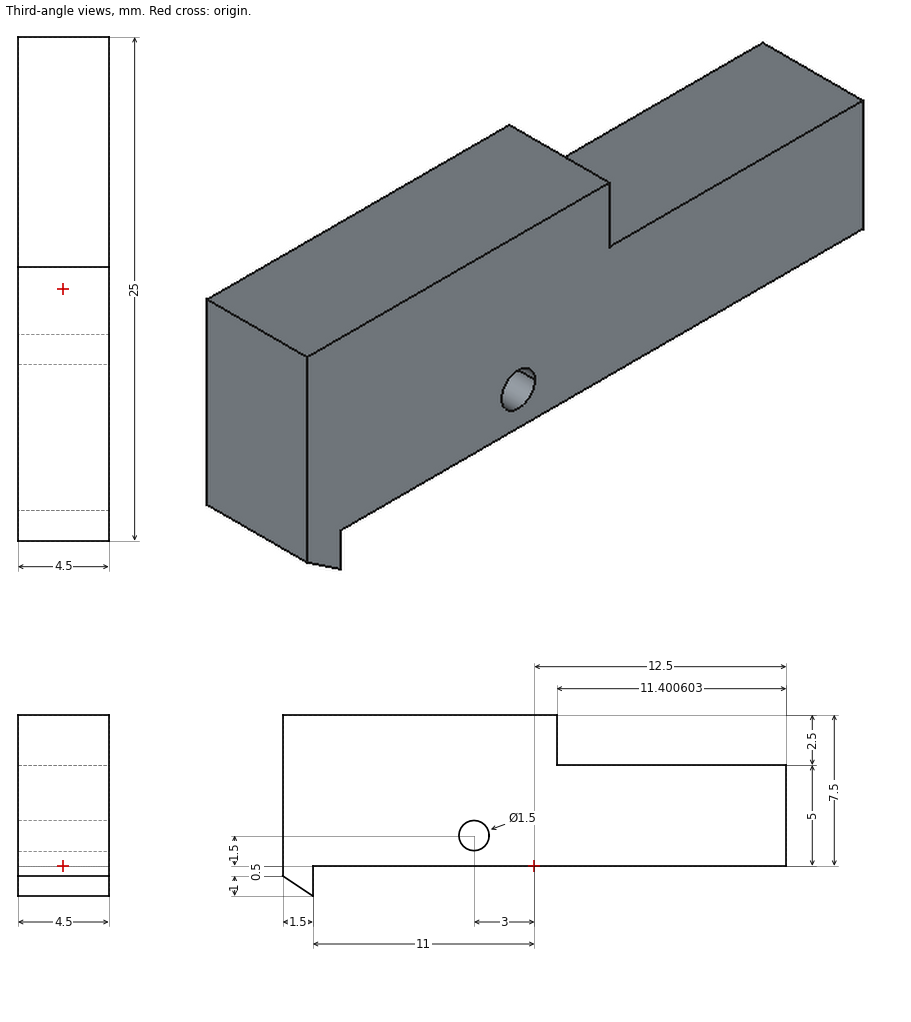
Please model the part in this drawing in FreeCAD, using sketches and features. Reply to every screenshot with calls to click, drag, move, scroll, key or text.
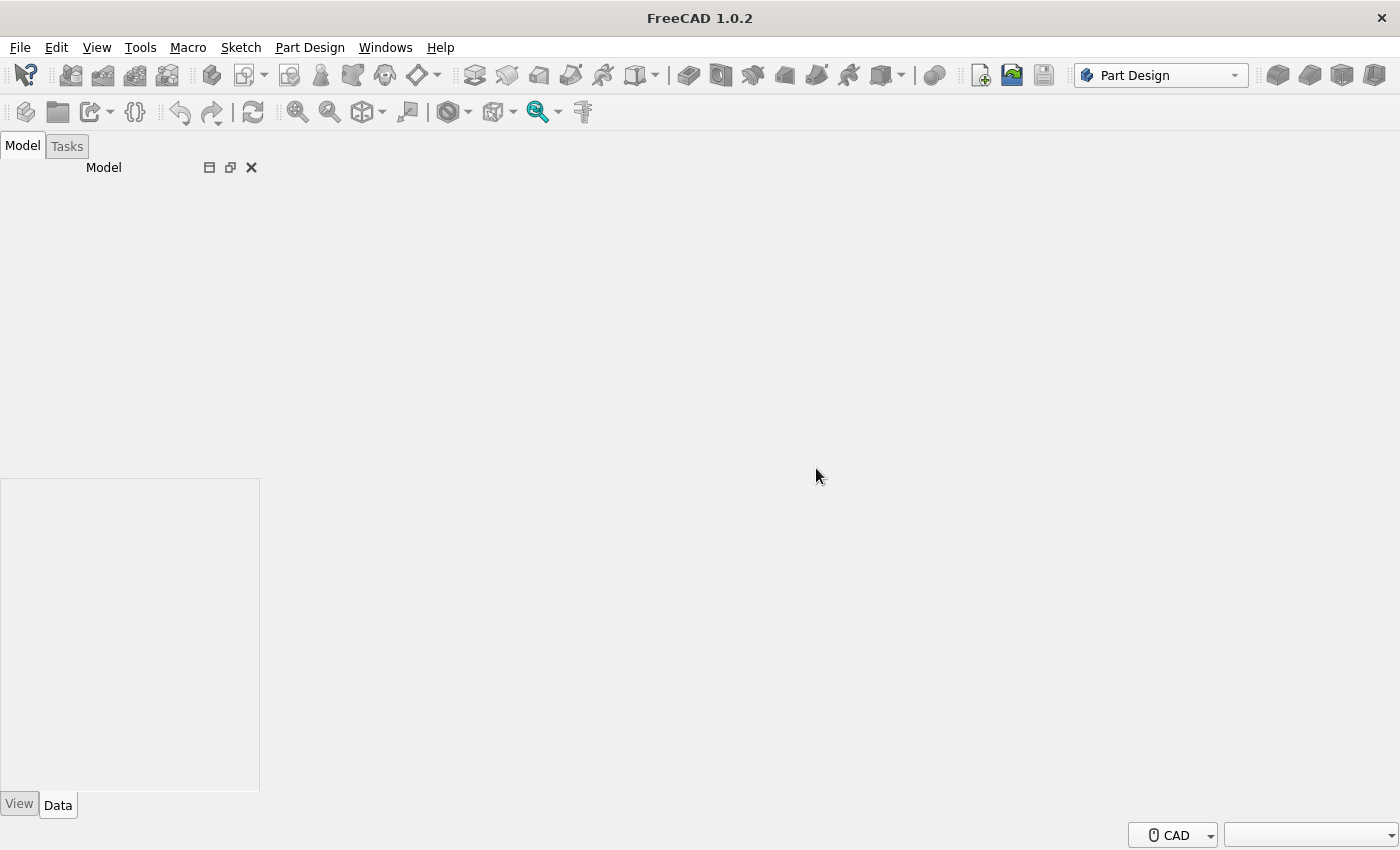
key(ctrl+n)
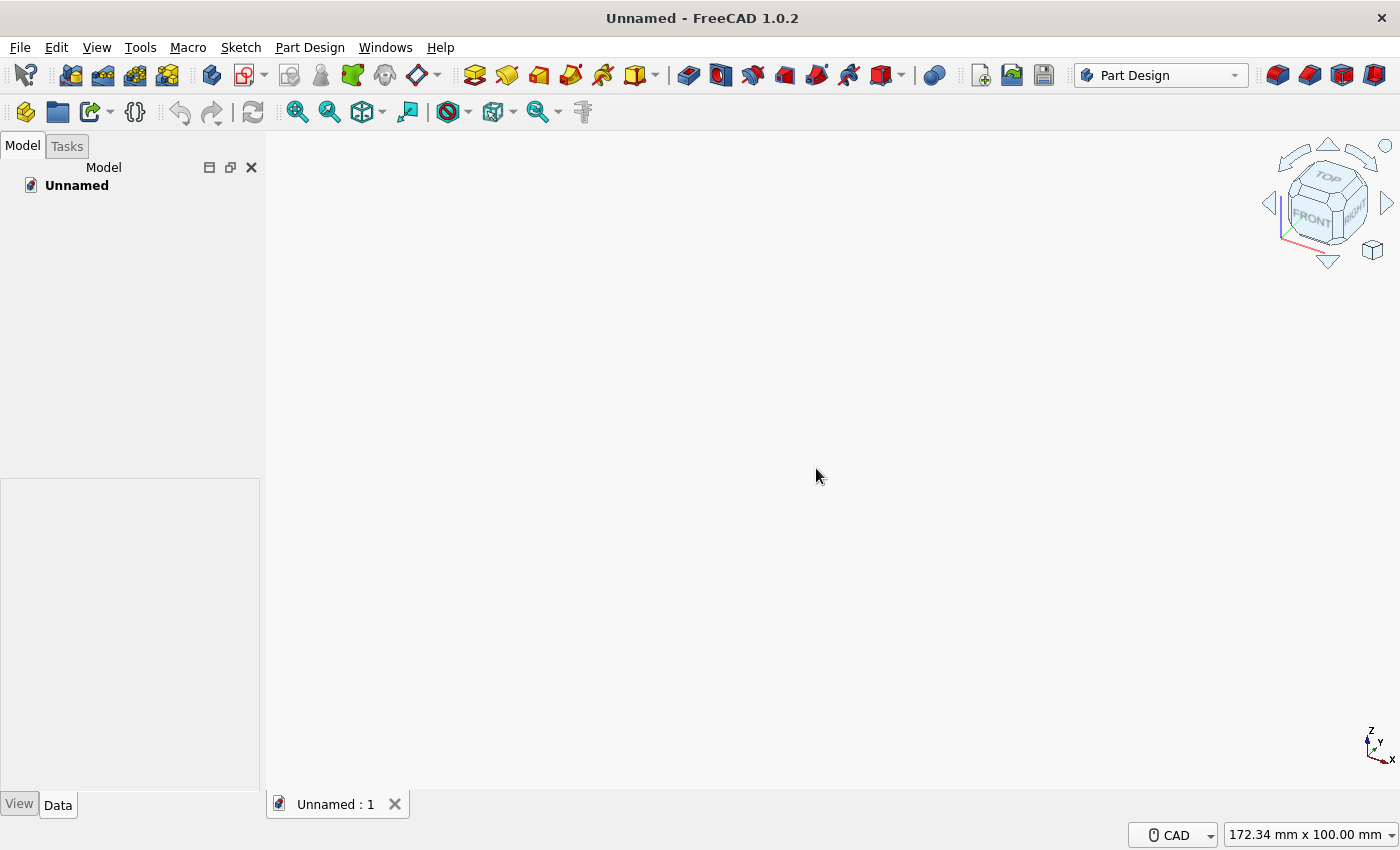
click(244, 76)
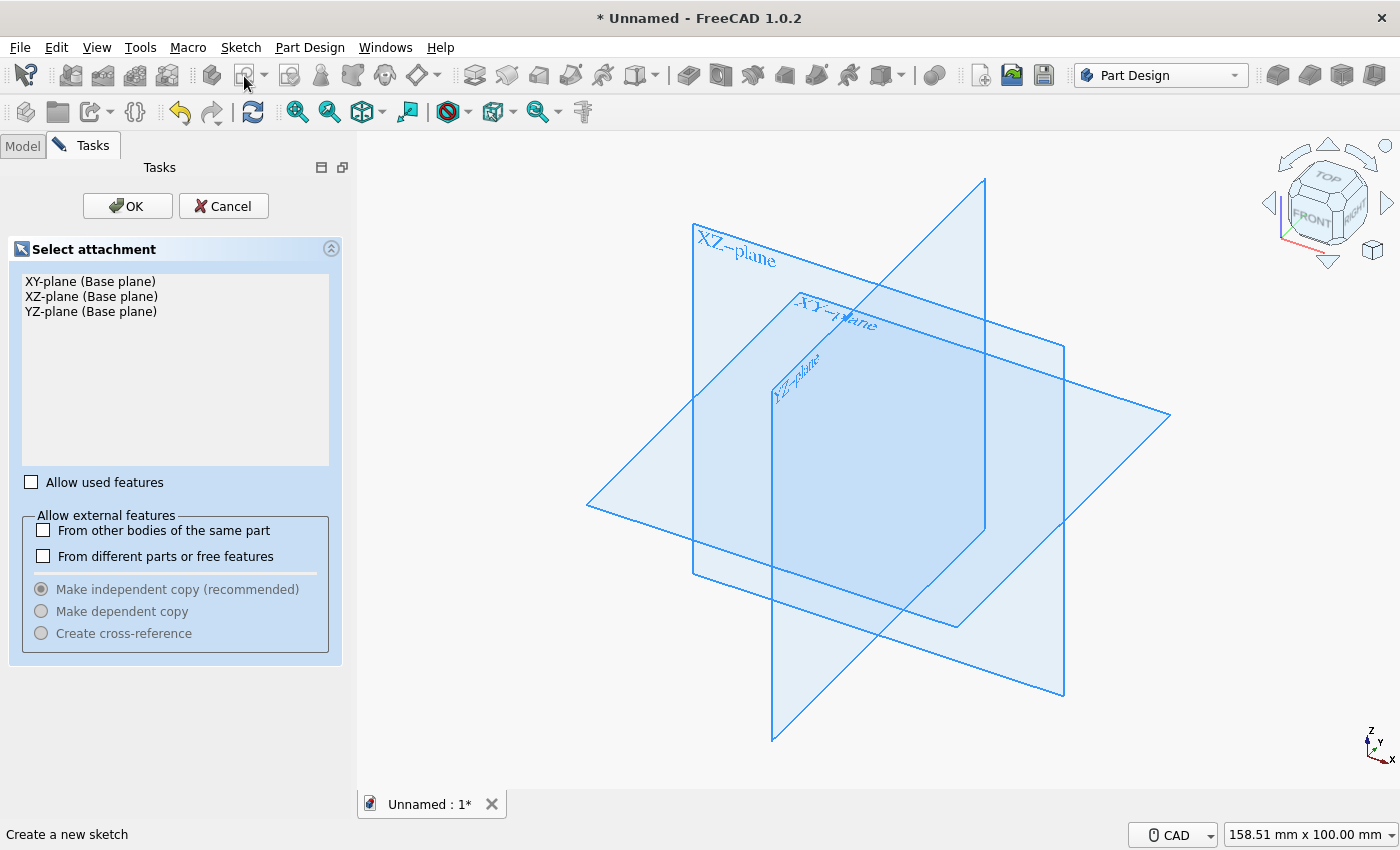
click(82, 282)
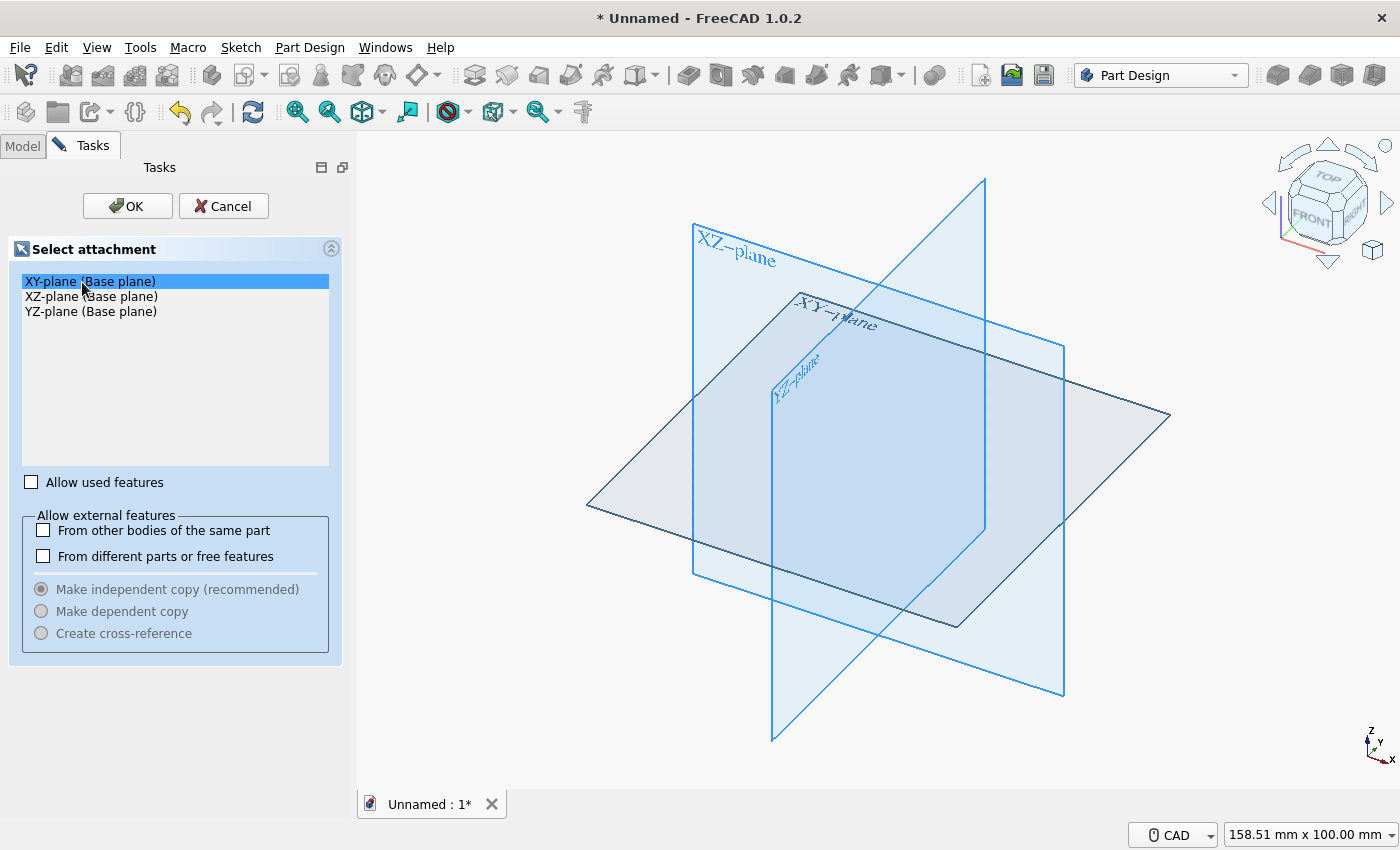
click(128, 206)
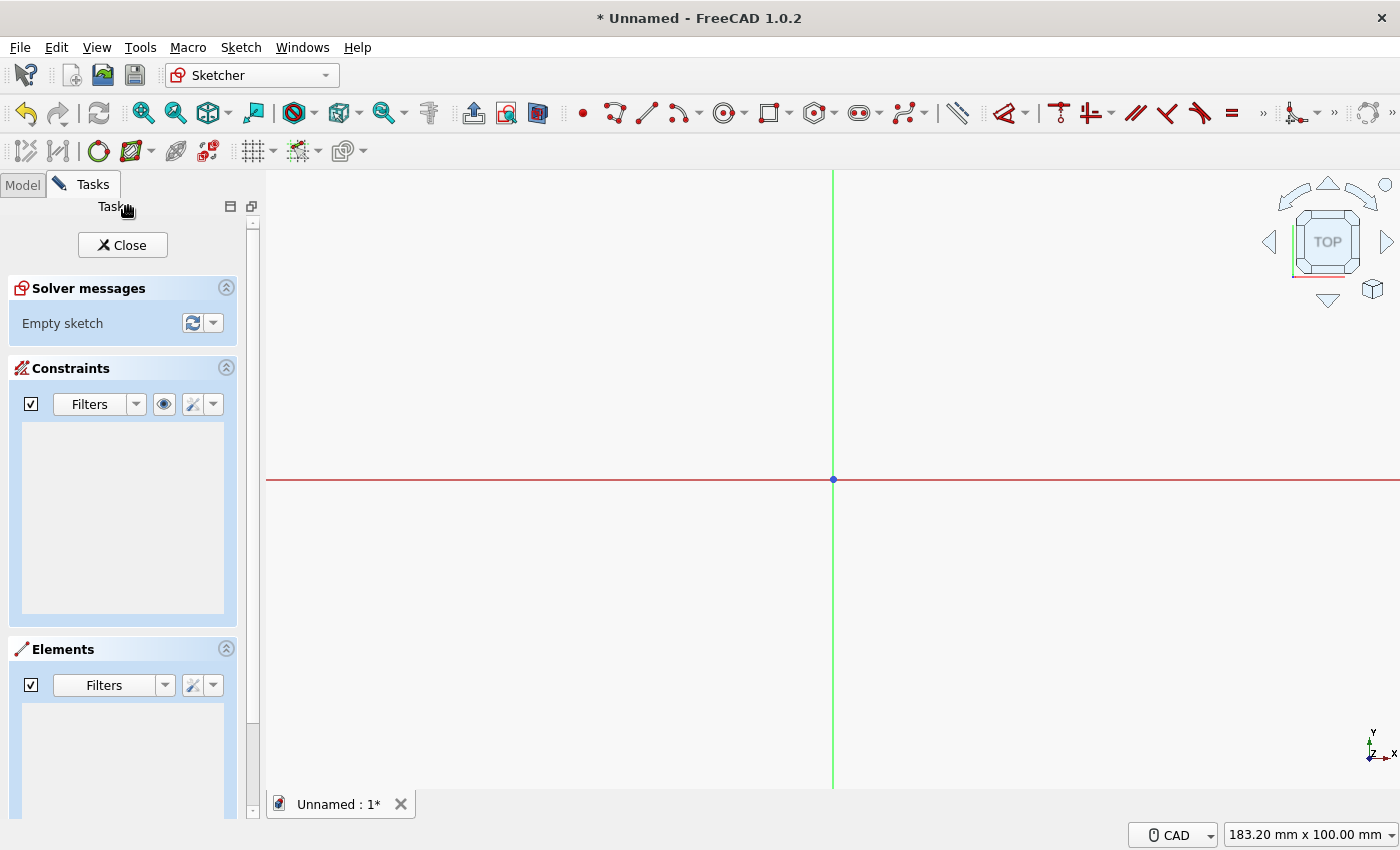
scroll(873, 480, up, 5)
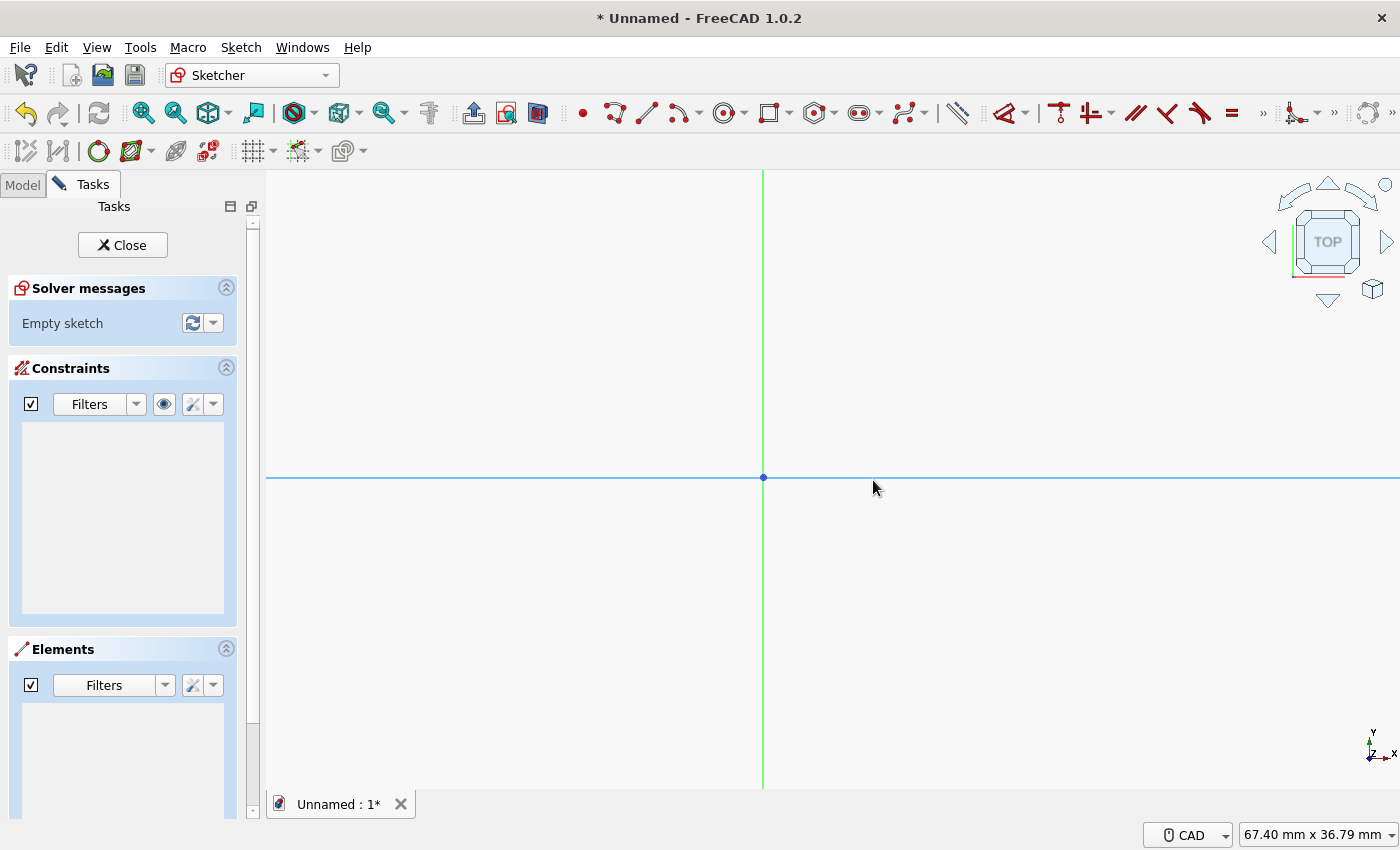
key(g)
key(v)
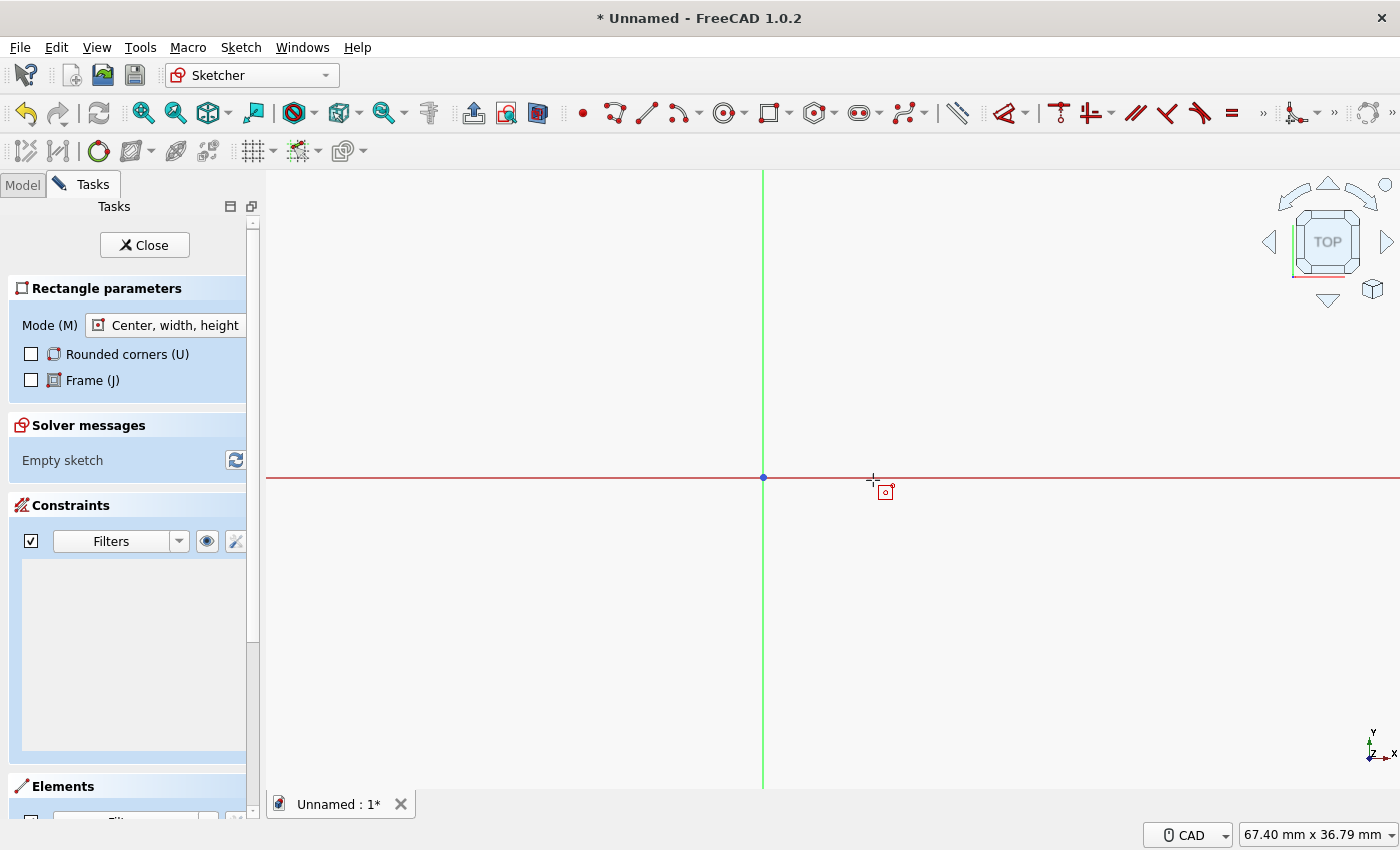
click(763, 478)
move(801, 267)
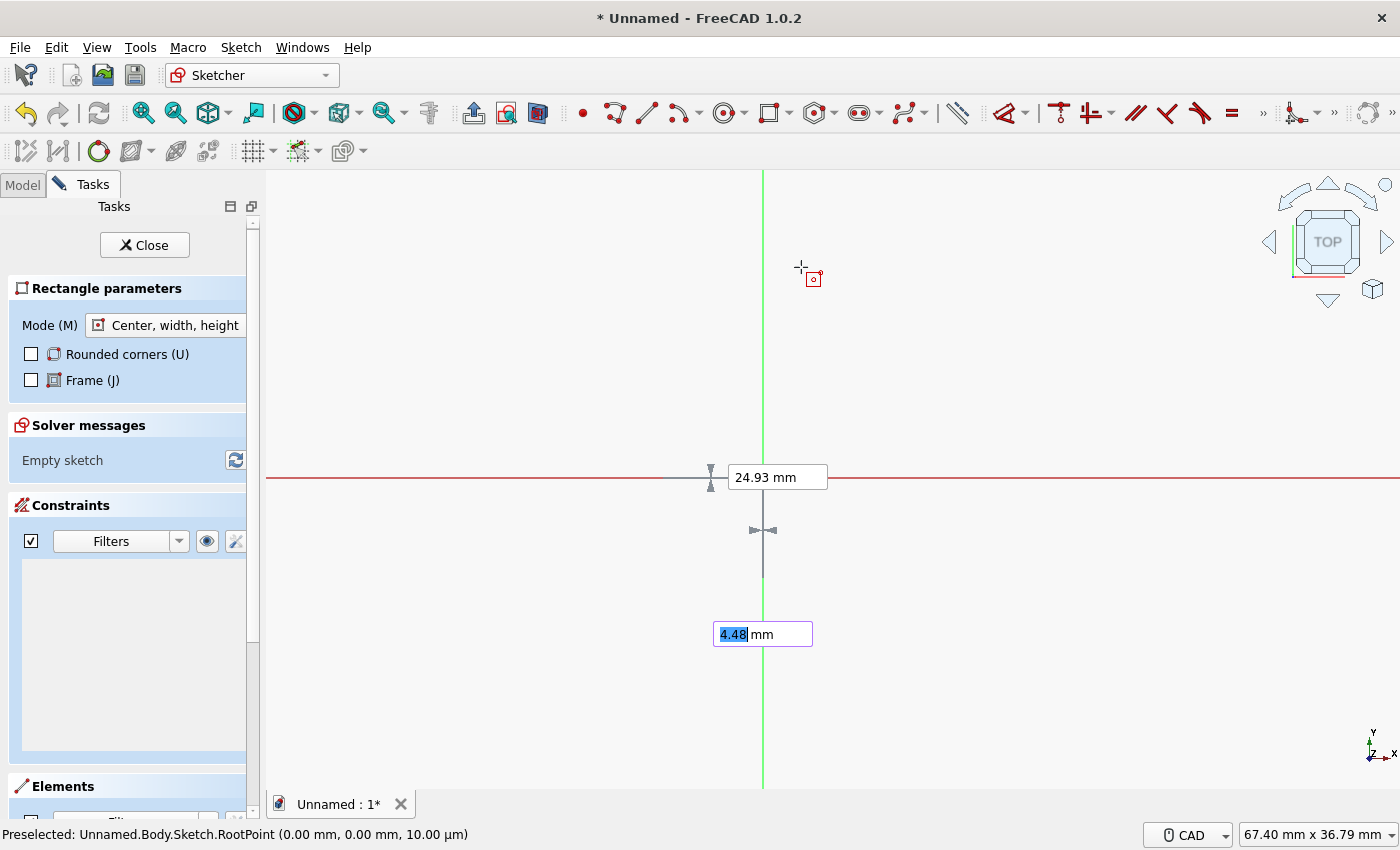
text(4.5)
key(Tab)
text(25)
key(Return)
key(Escape)